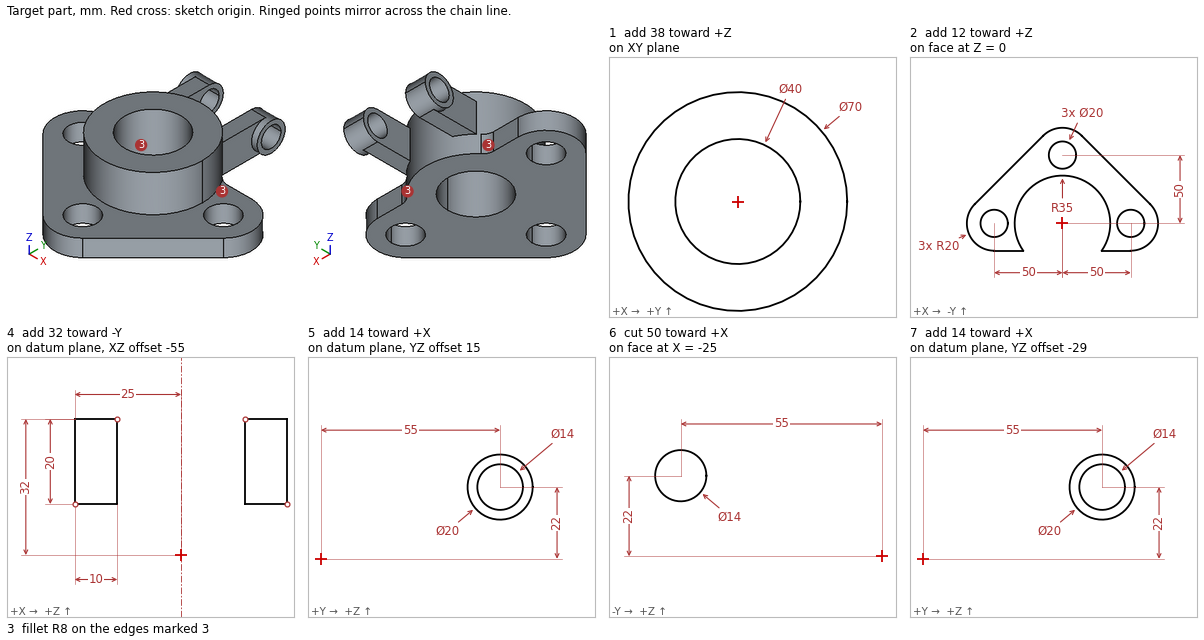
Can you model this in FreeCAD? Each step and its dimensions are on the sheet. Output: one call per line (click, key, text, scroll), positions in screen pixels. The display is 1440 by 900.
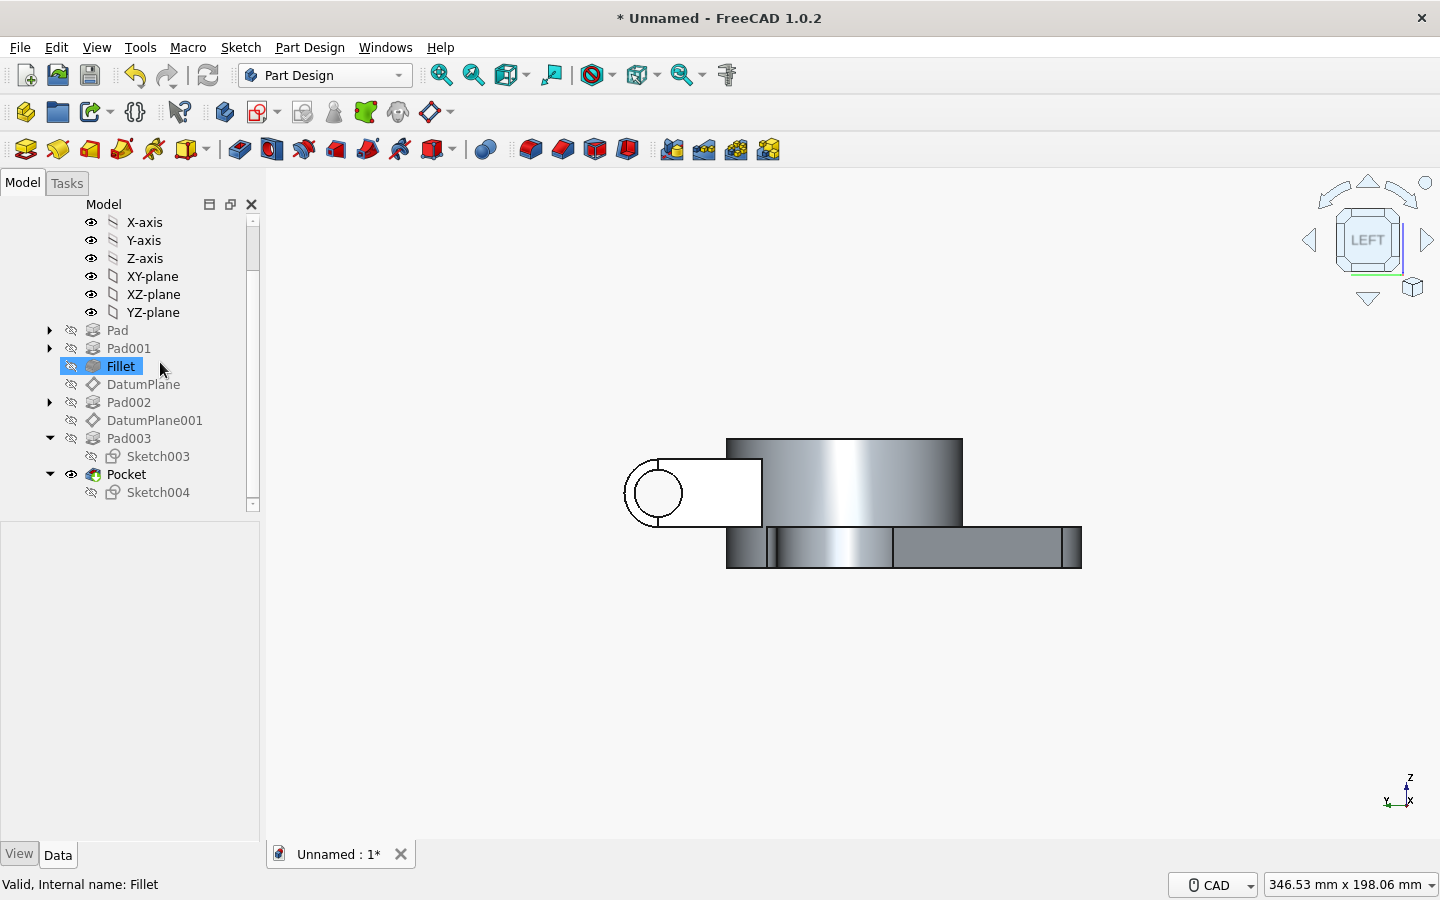
scroll(160, 362, up, 15)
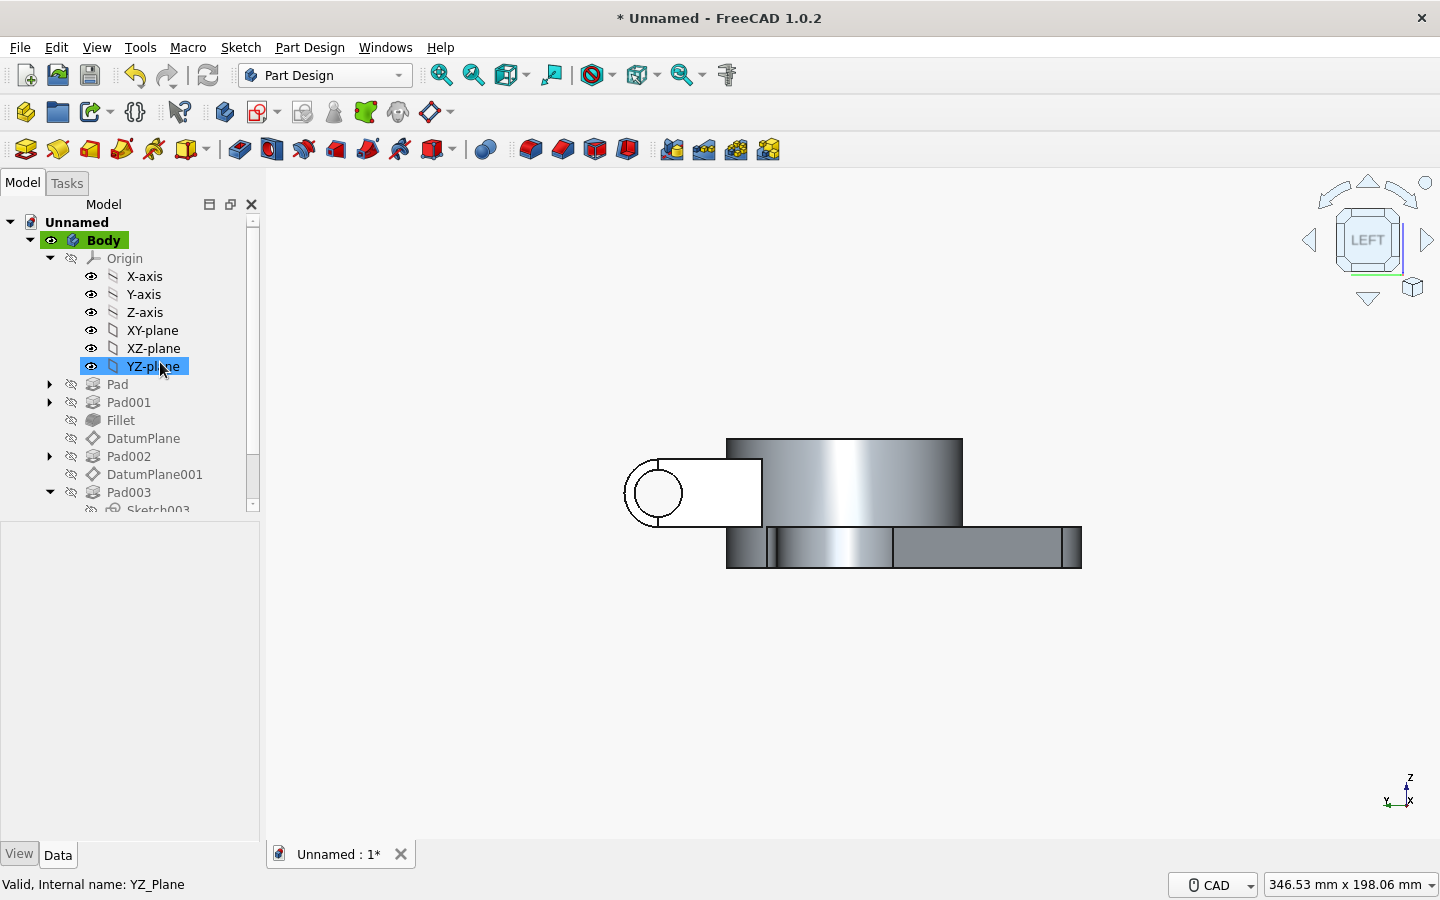
click(136, 366)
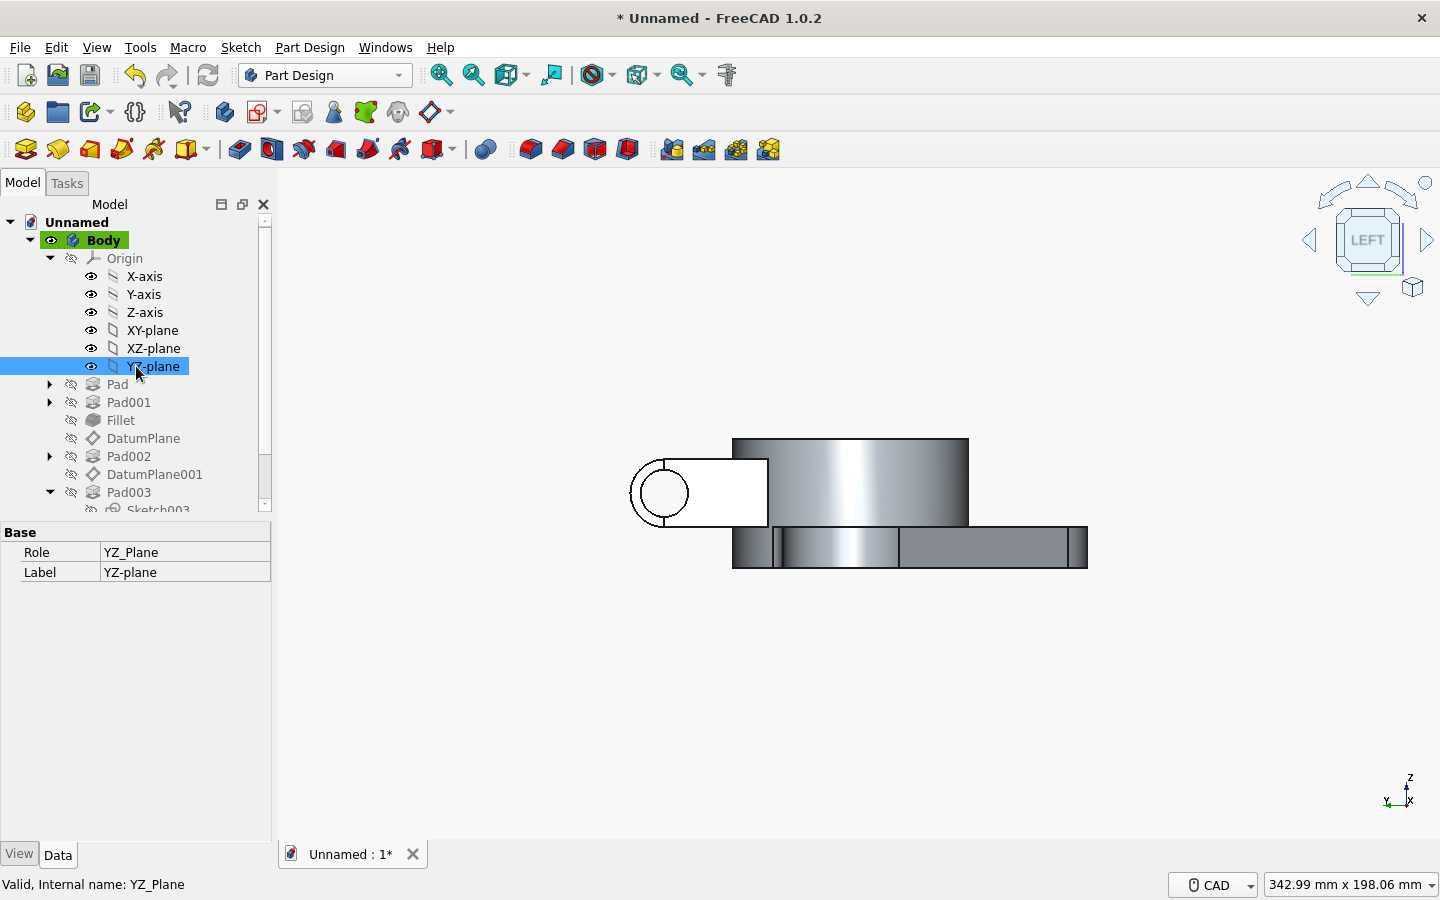
click(430, 112)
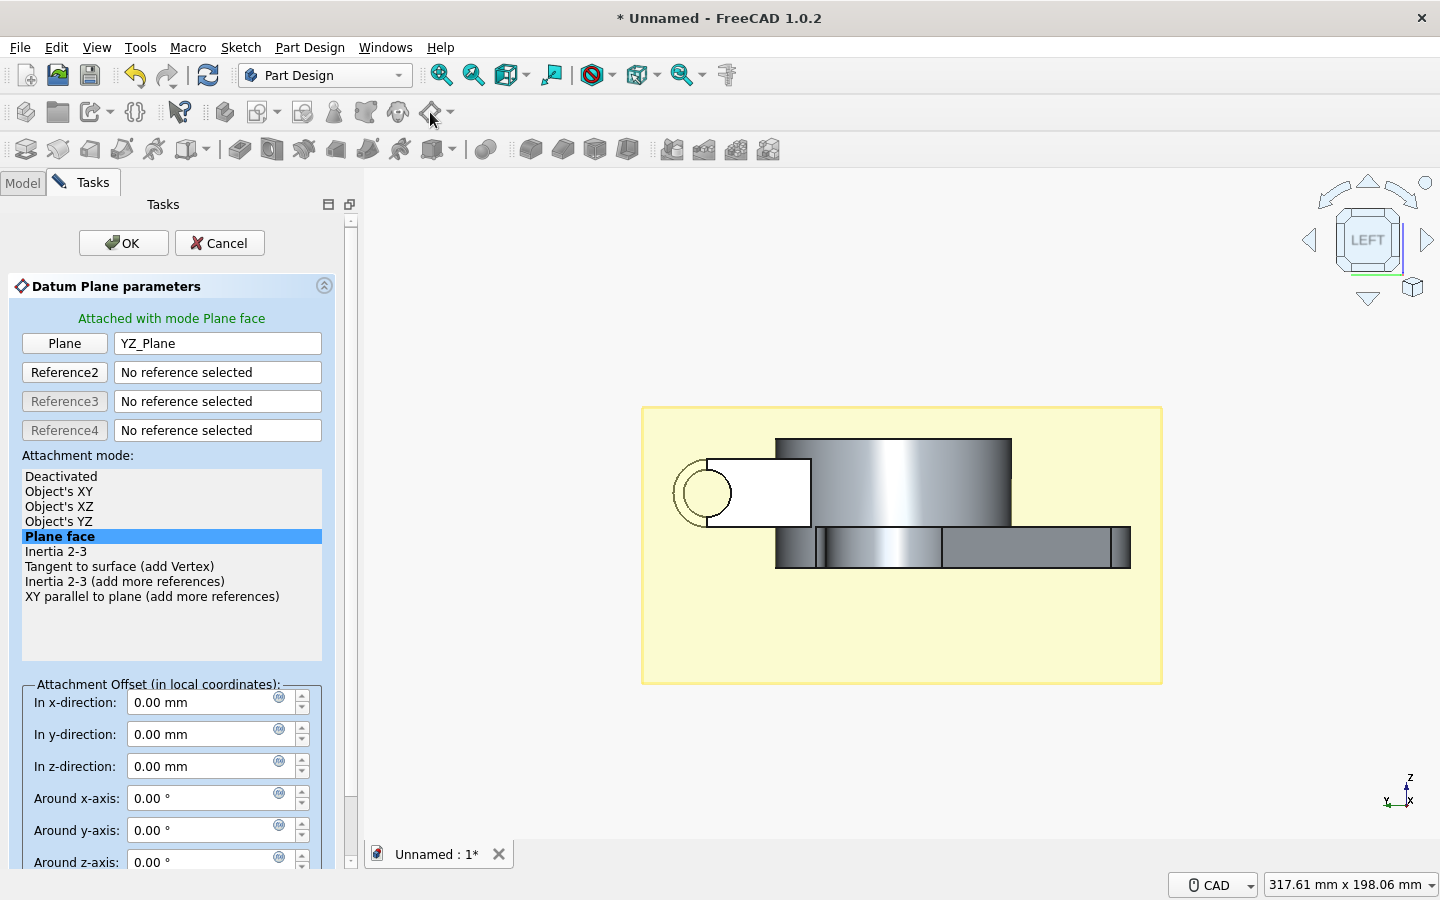
triple_click(210, 766)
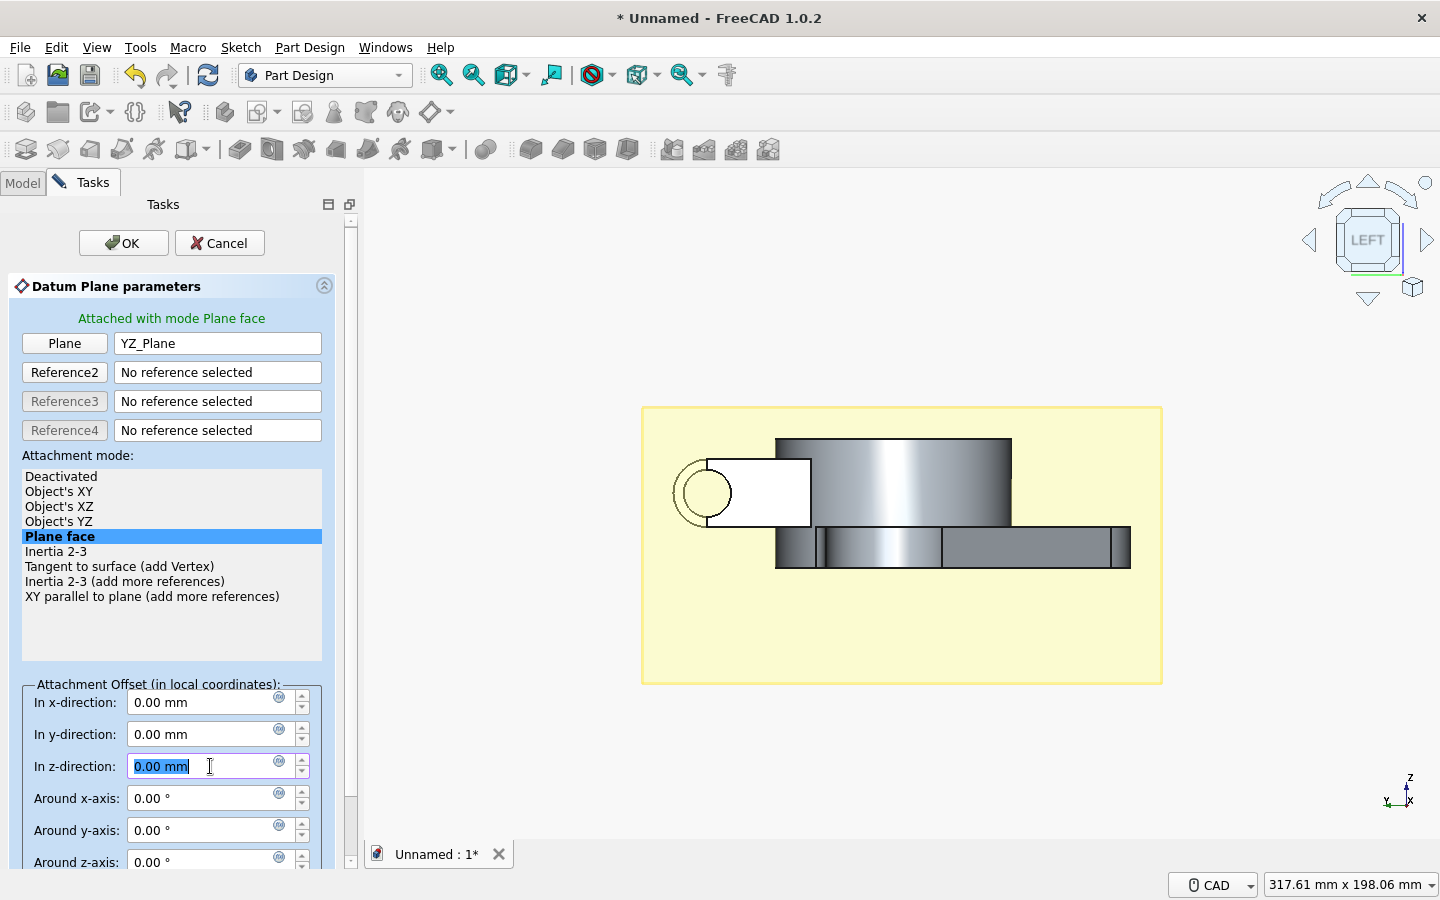
text(-29)
key(Tab)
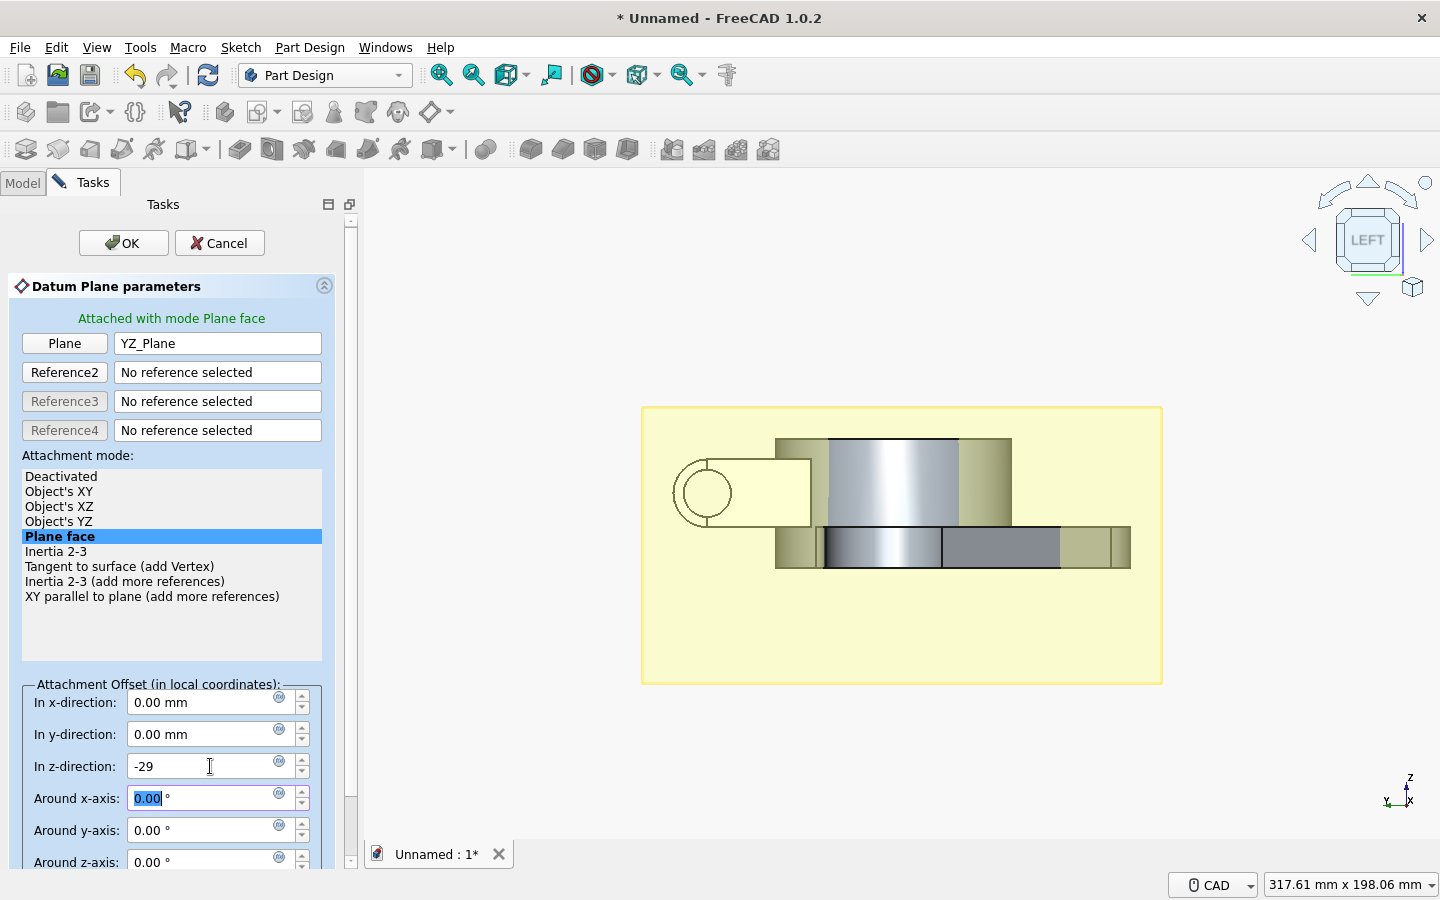
click(124, 243)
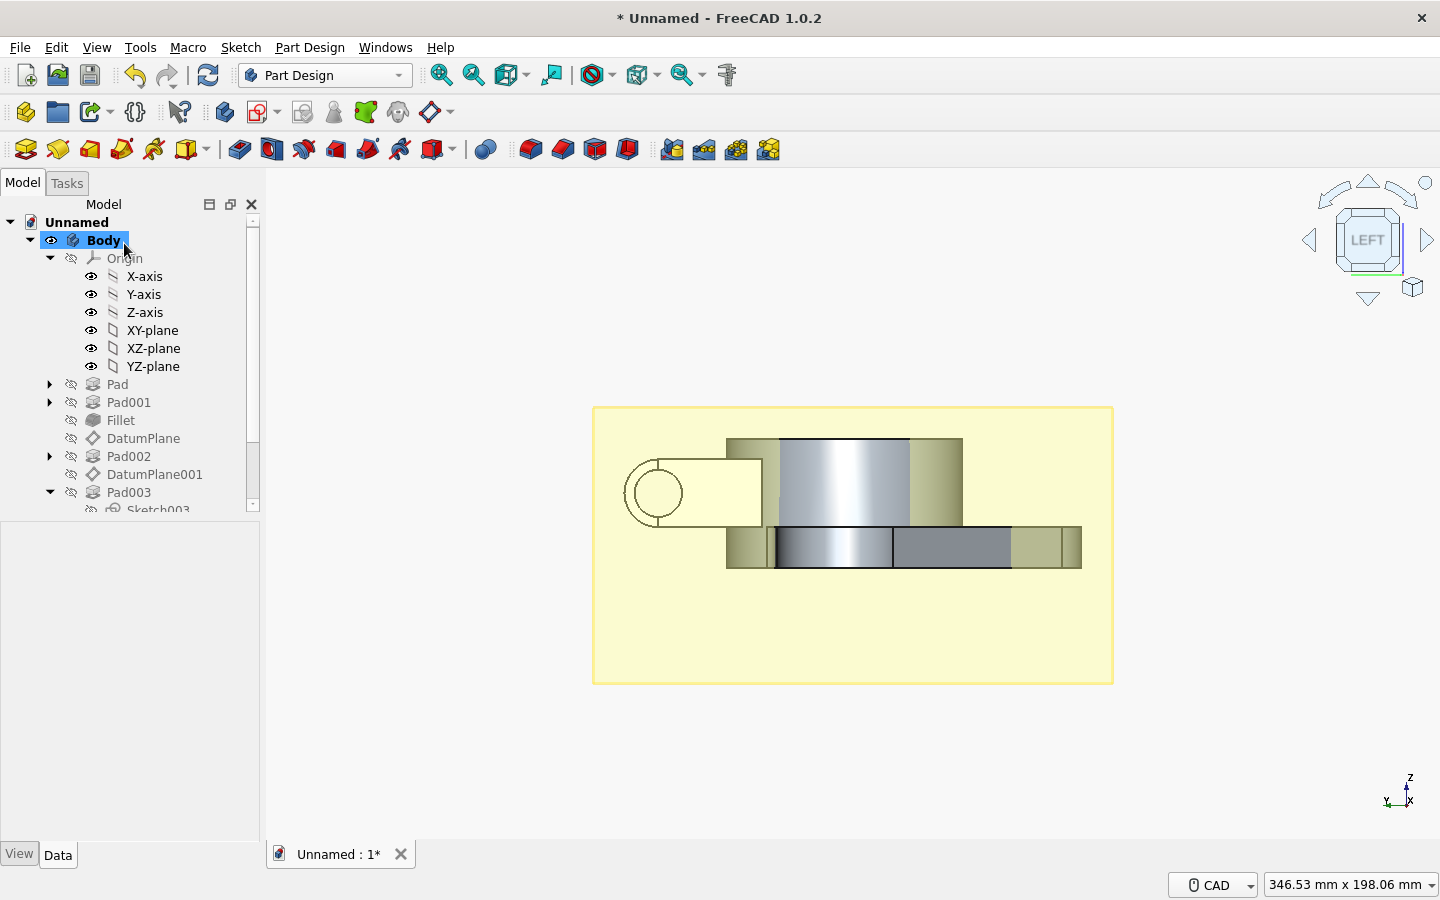
scroll(100, 362, down, 3)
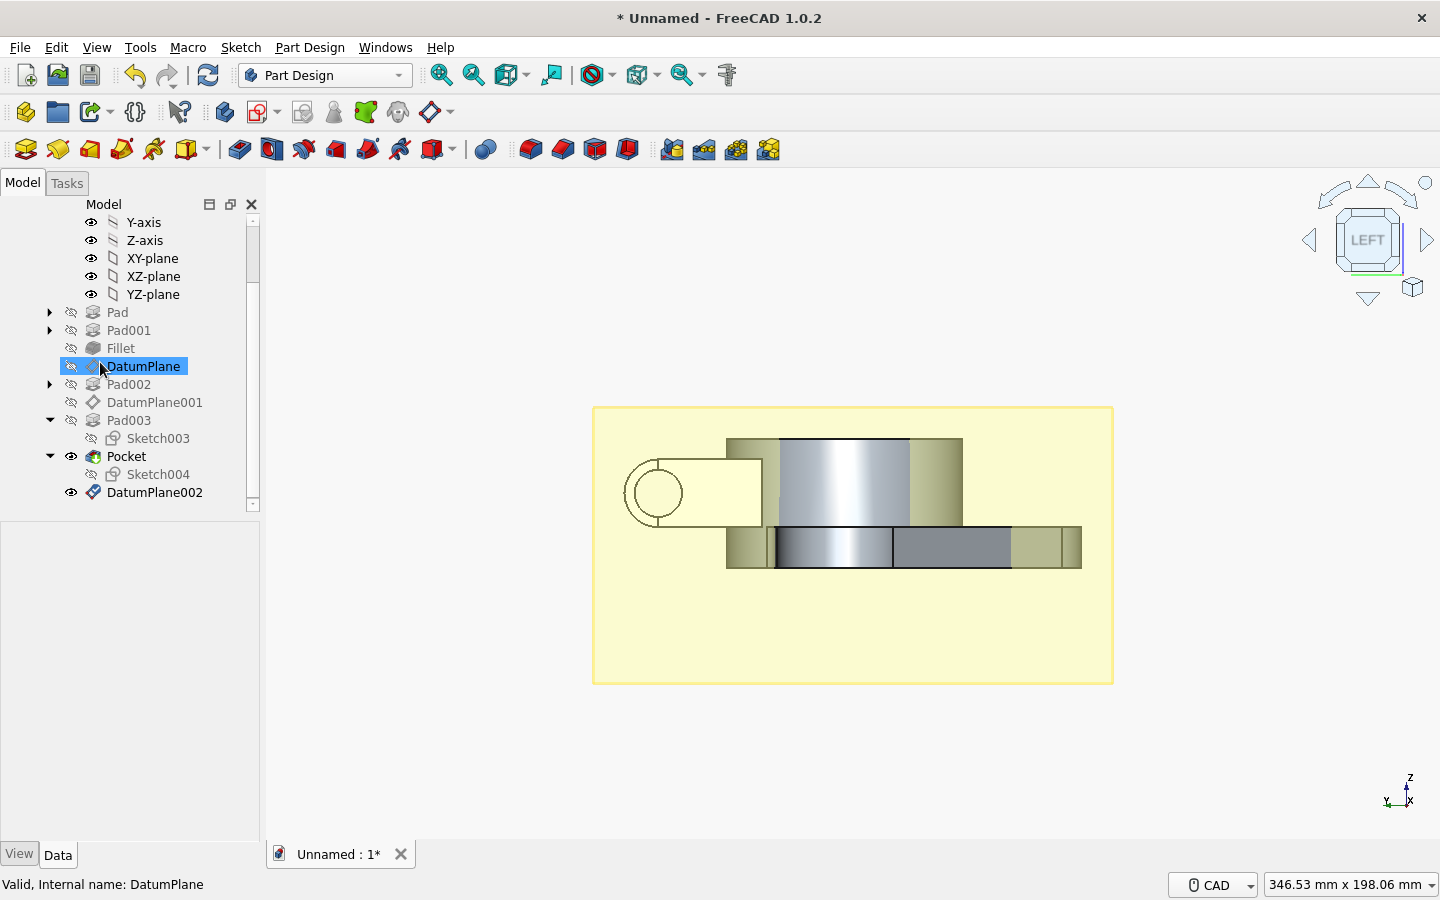
click(116, 492)